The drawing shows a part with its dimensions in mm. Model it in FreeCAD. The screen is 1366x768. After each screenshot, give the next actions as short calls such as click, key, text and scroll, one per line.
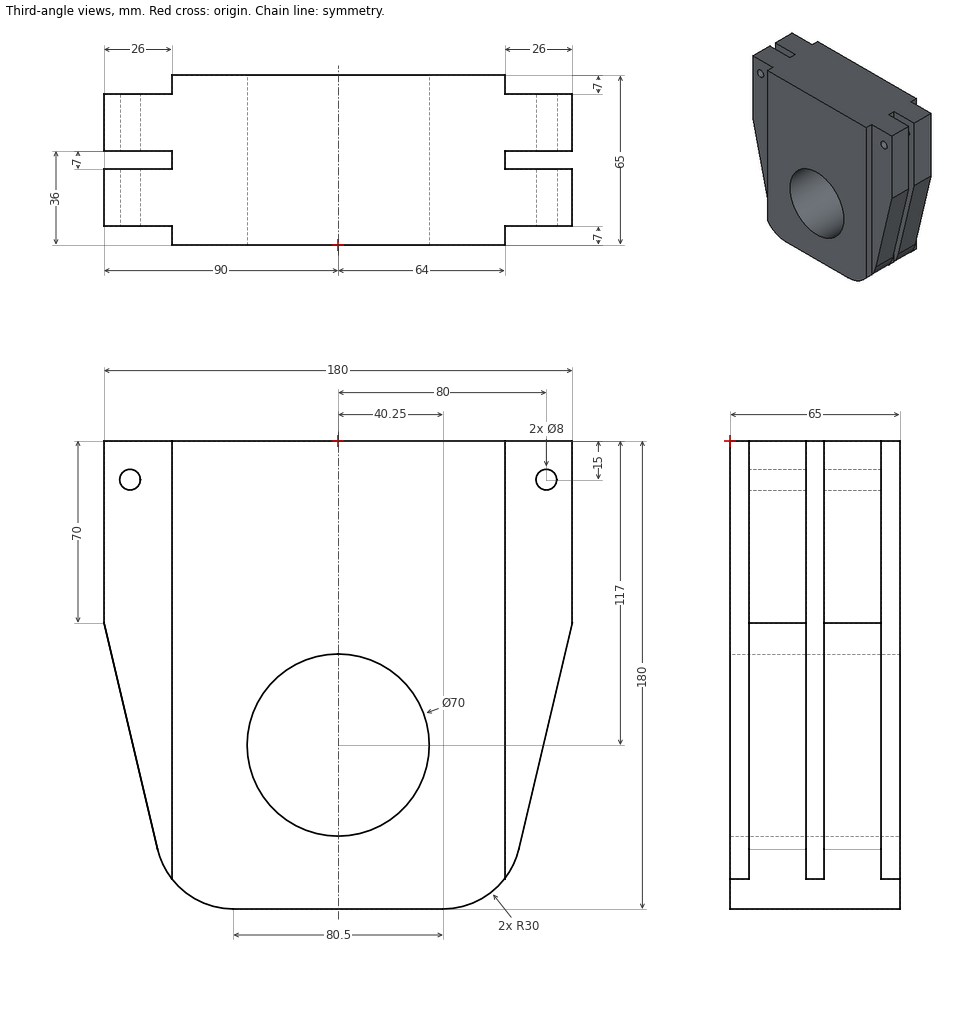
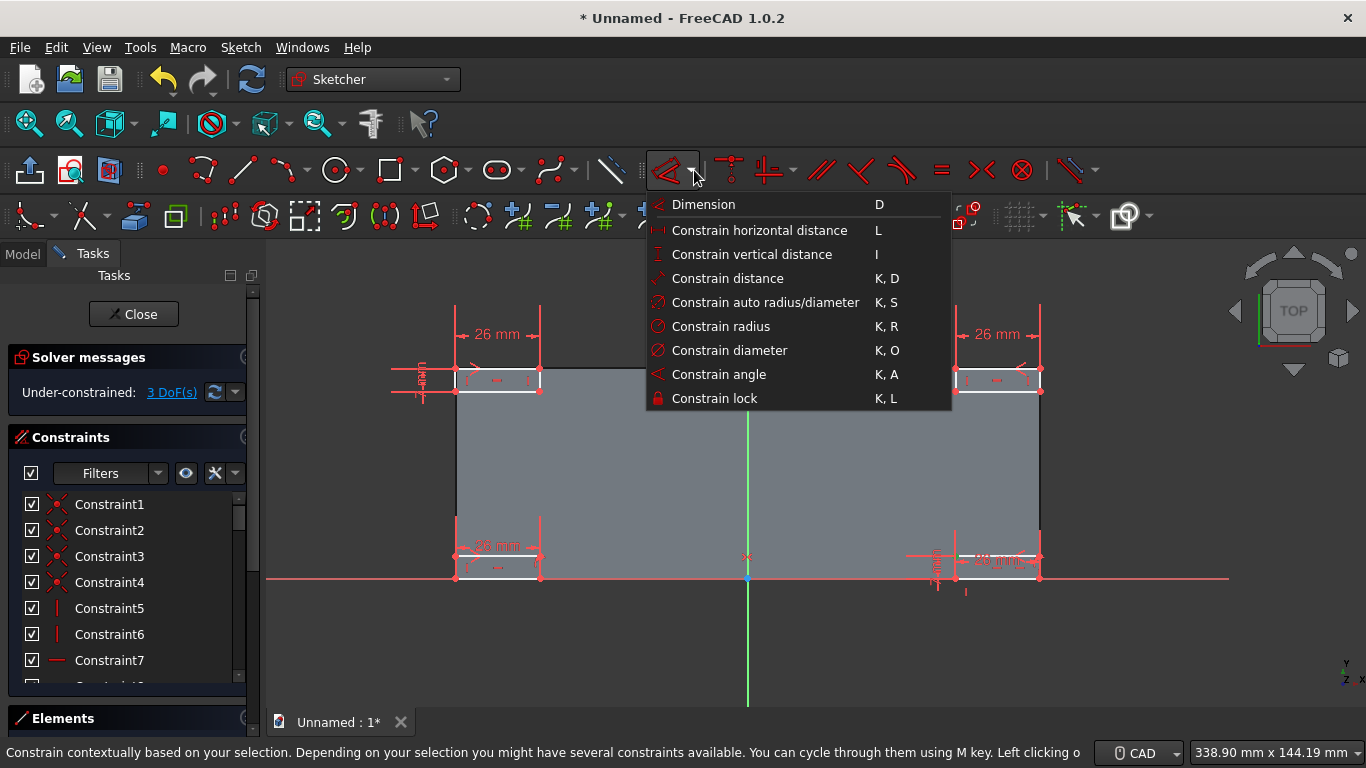
click(799, 230)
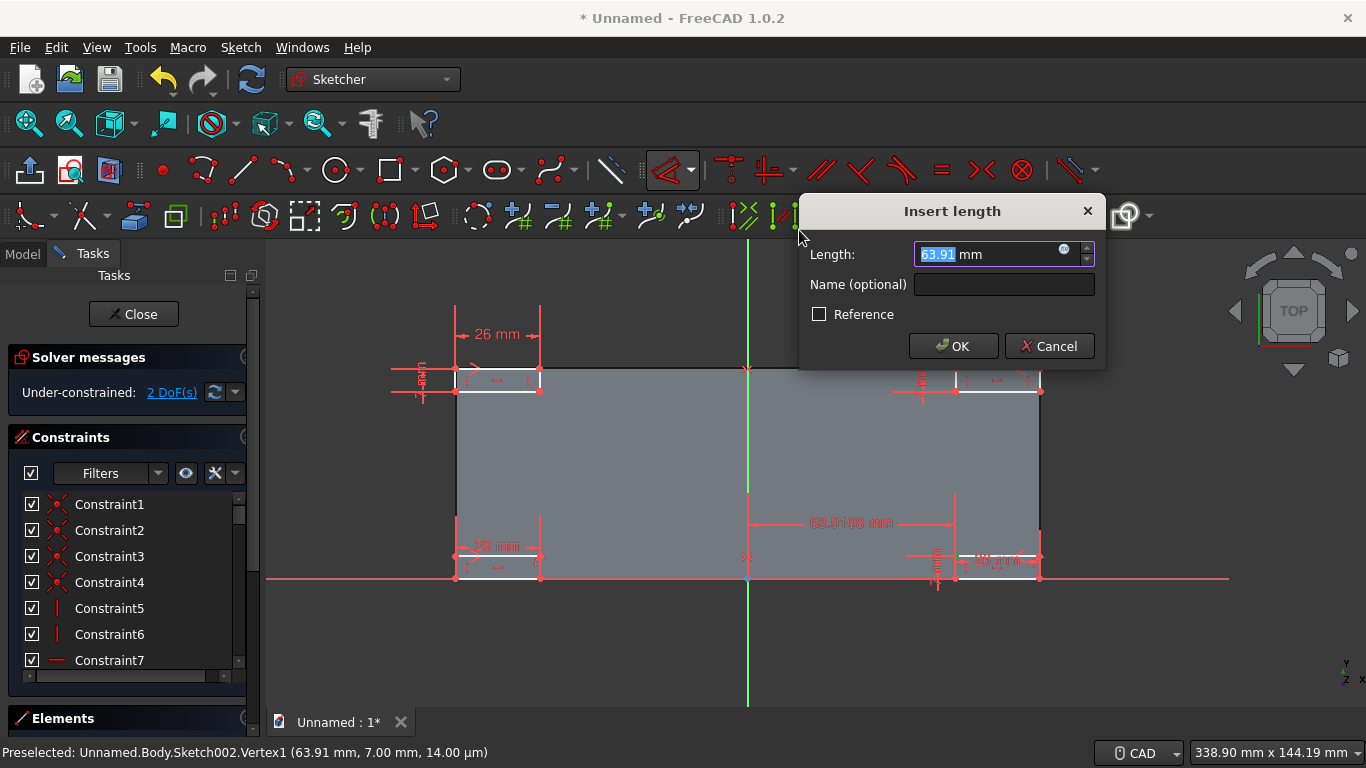
text(64)
key(Return)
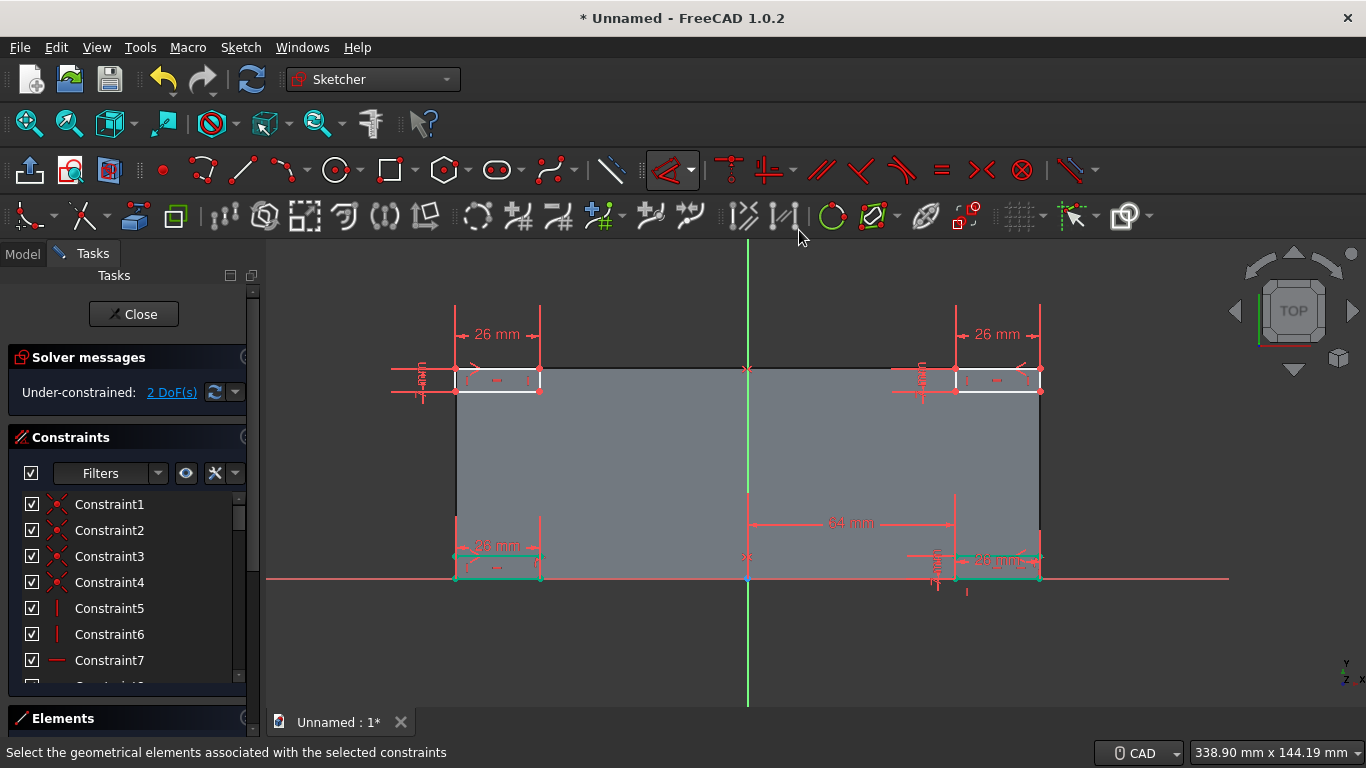
click(956, 369)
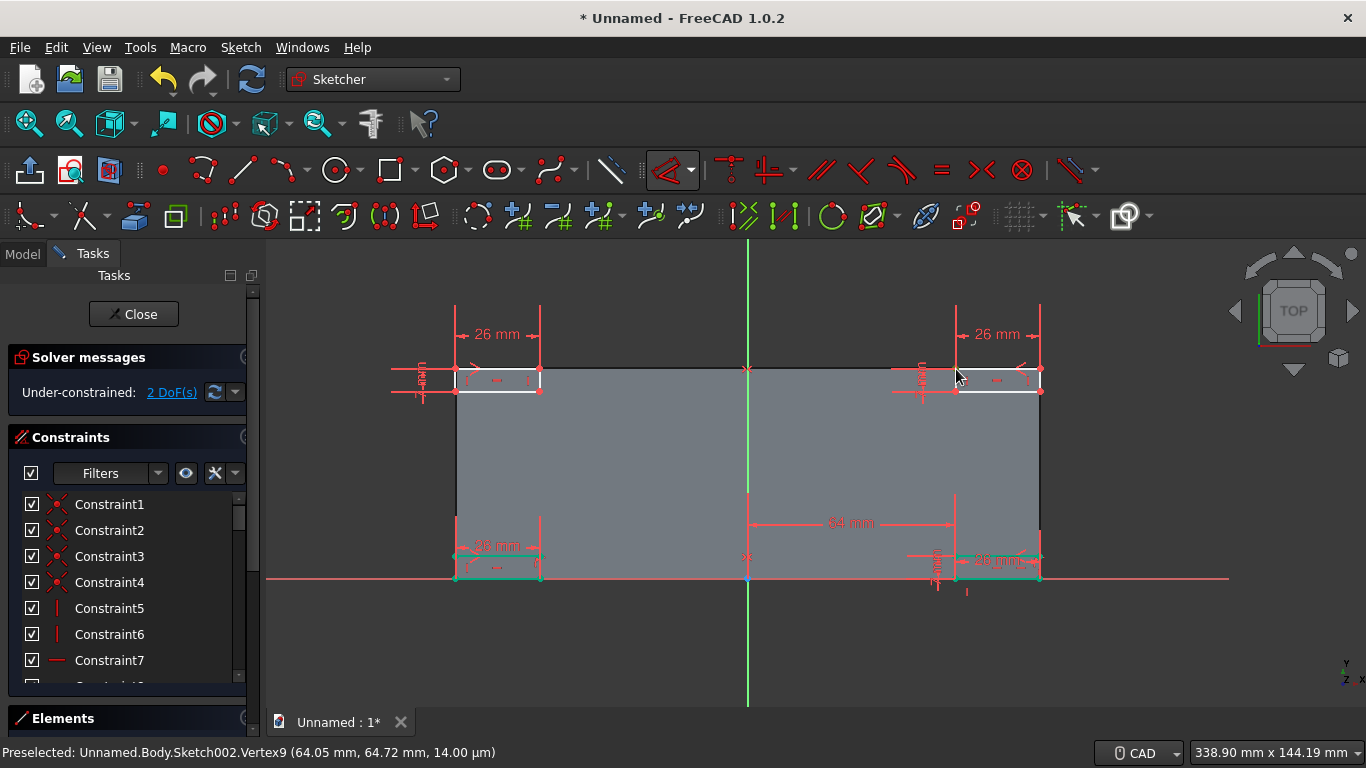
click(694, 170)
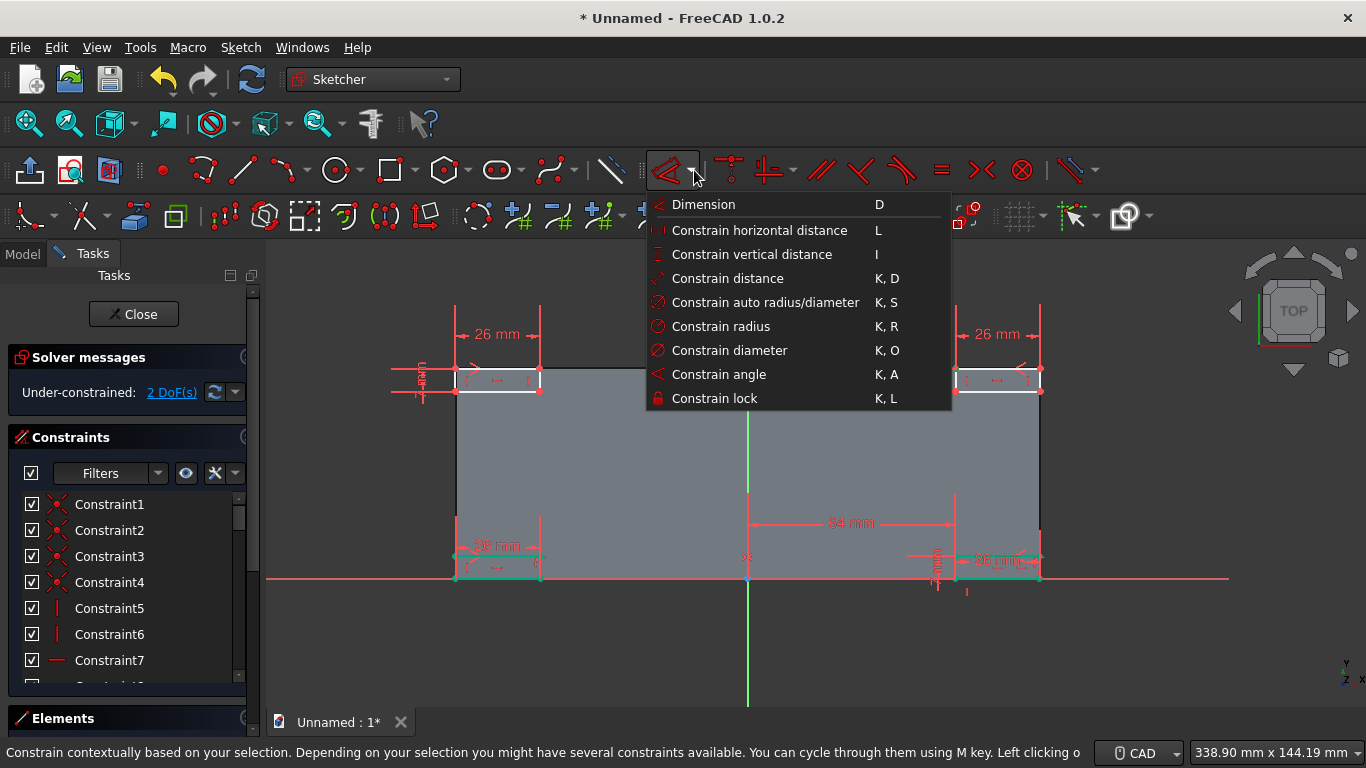
click(799, 230)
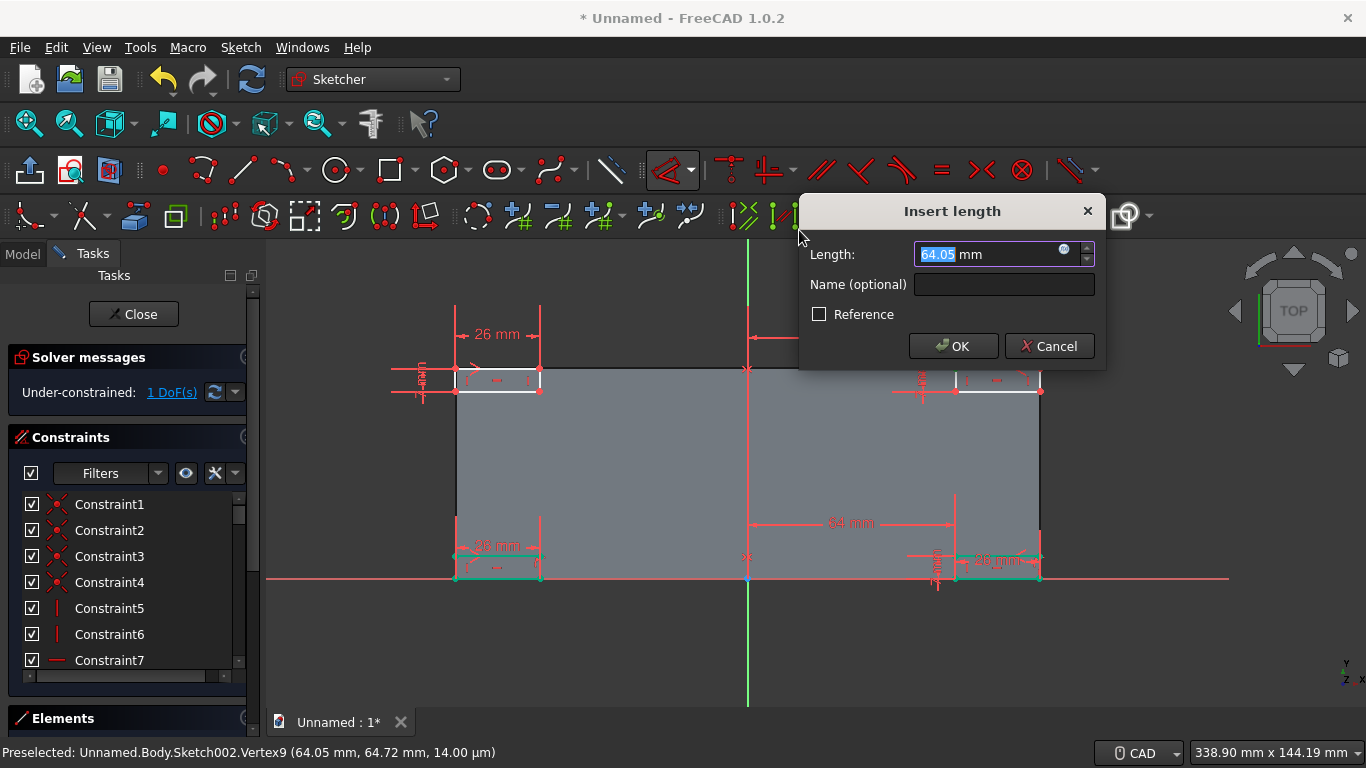
text(64)
key(Return)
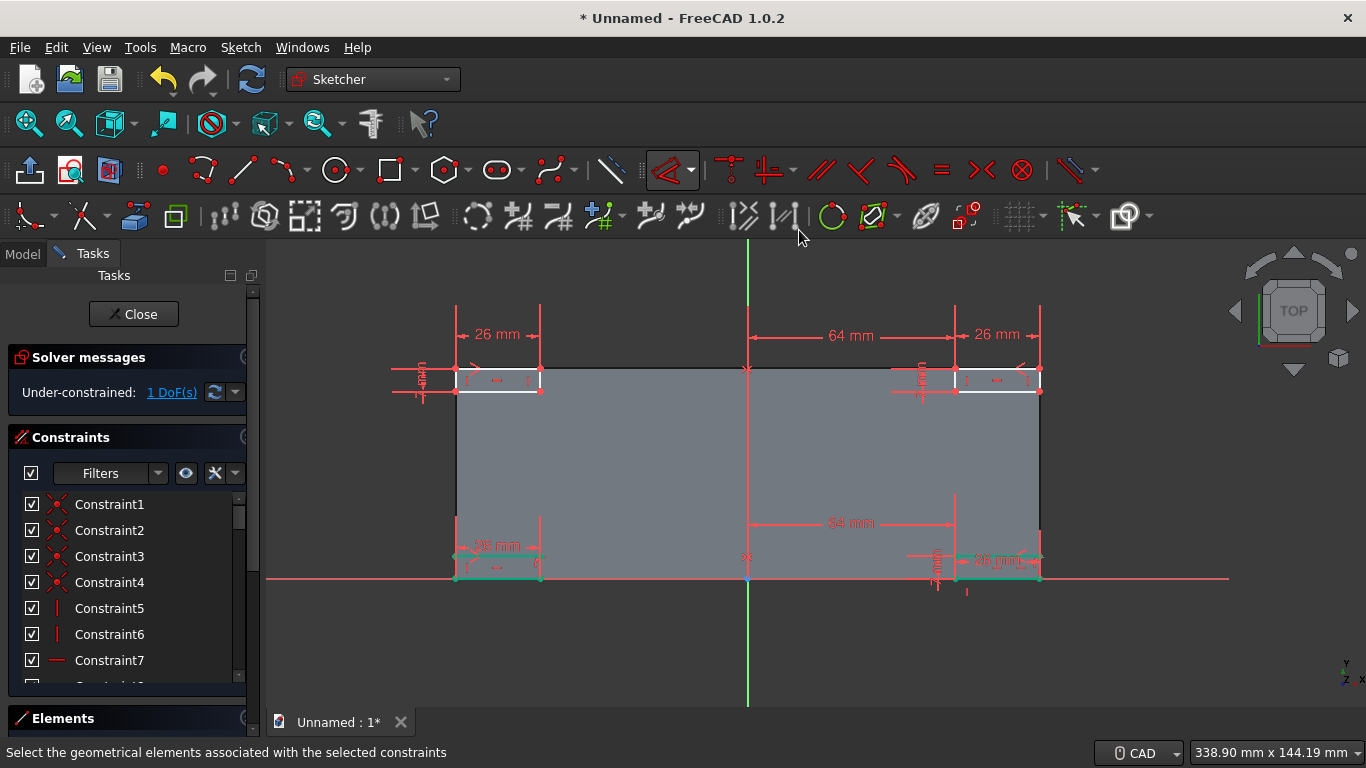
click(955, 369)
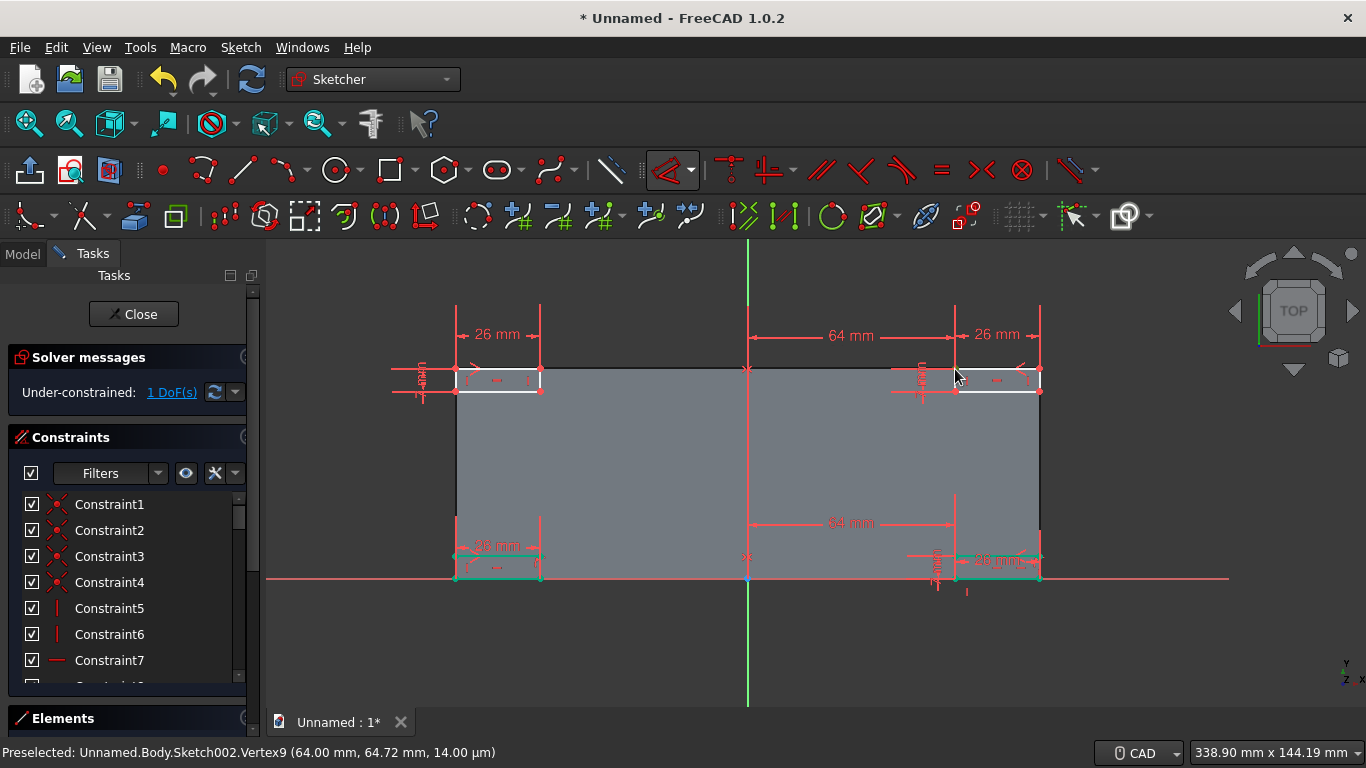
click(694, 170)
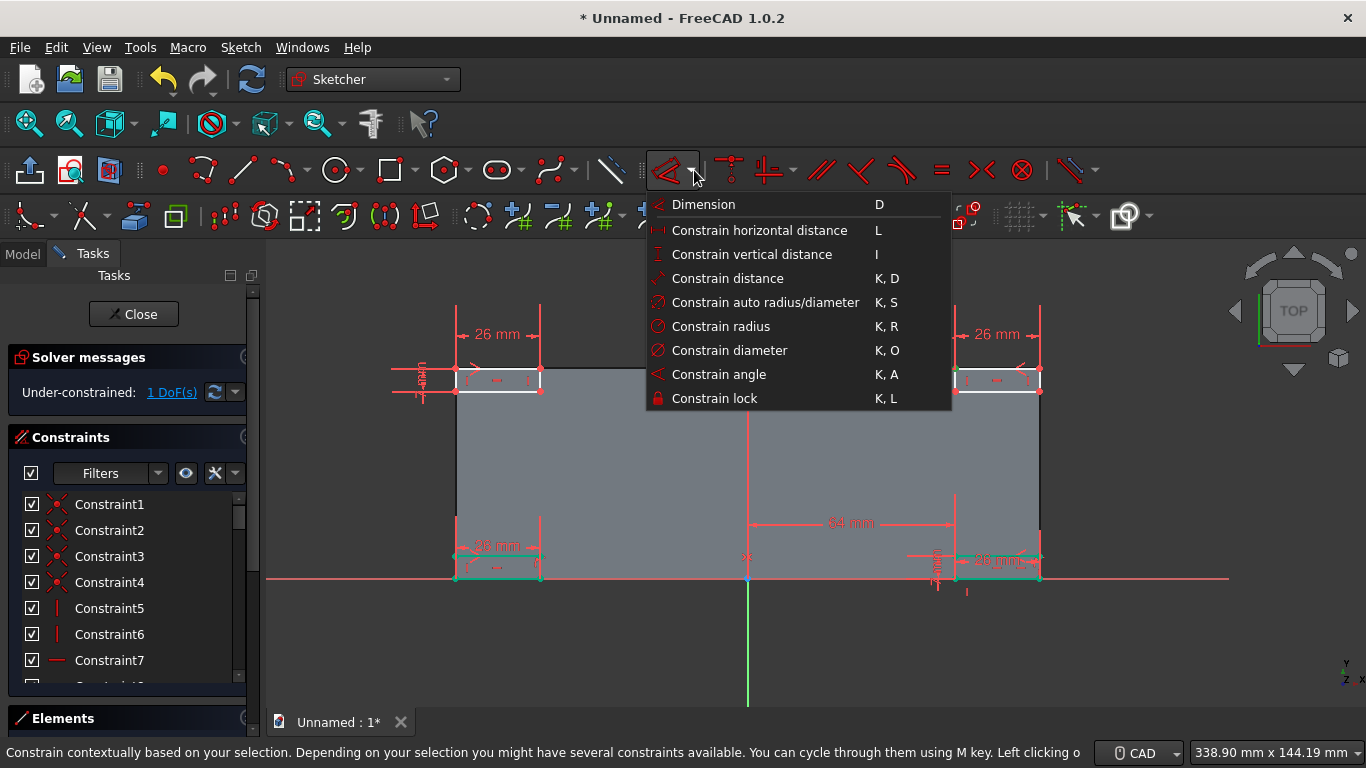
click(799, 254)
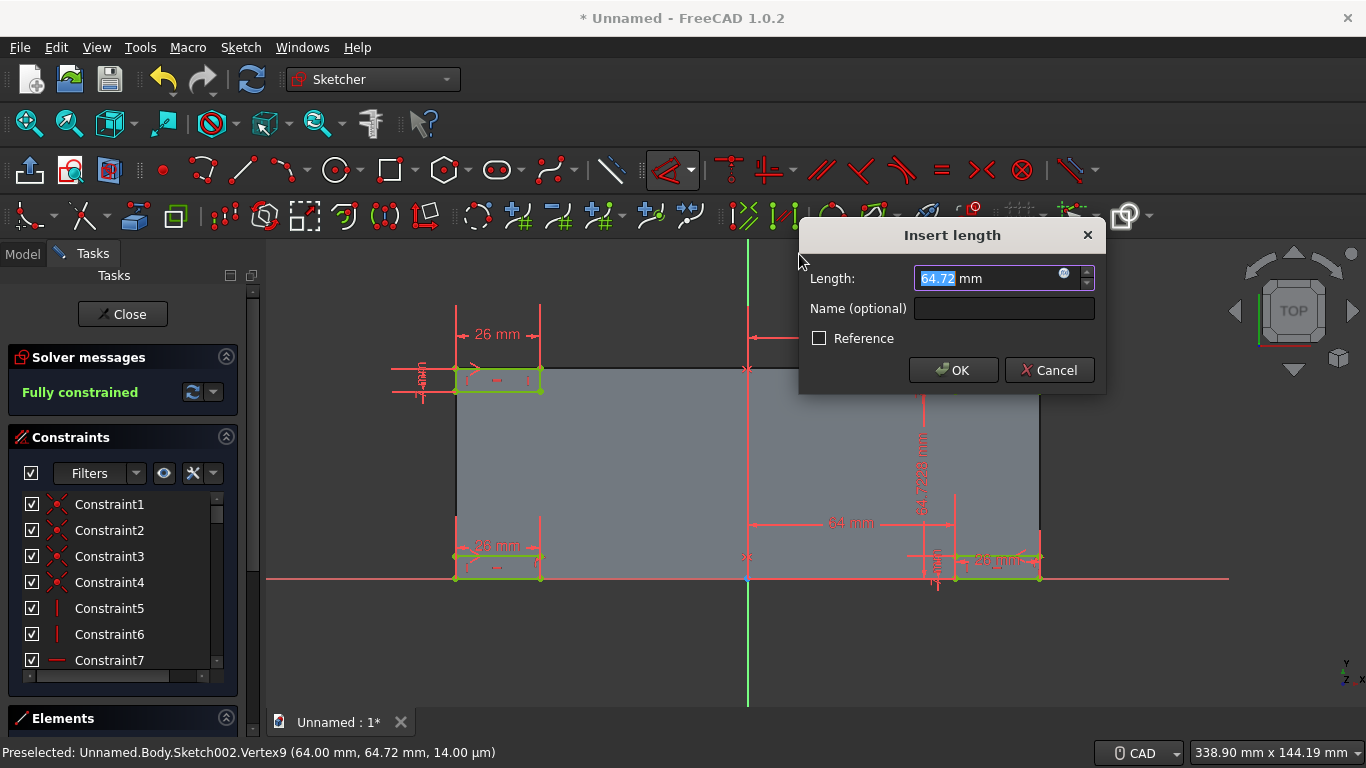
text(65)
key(Return)